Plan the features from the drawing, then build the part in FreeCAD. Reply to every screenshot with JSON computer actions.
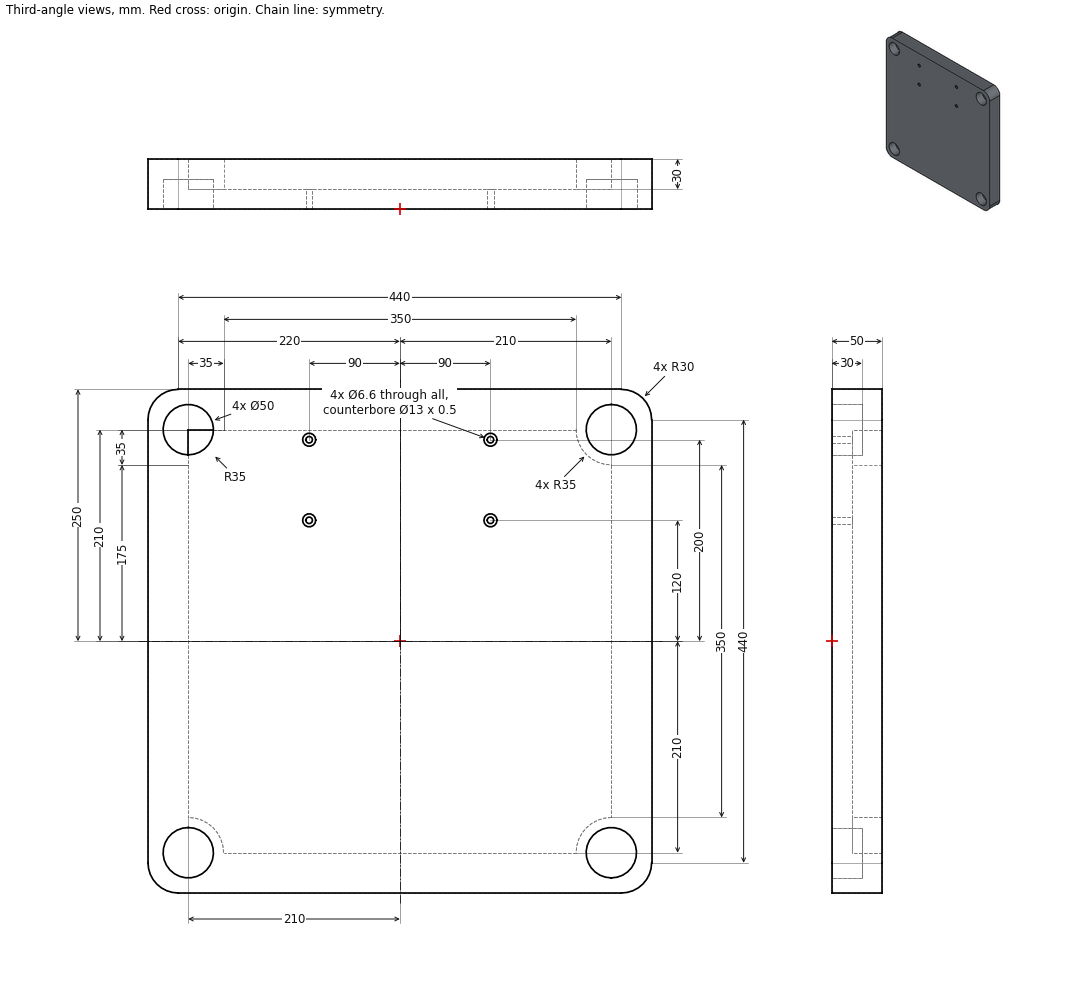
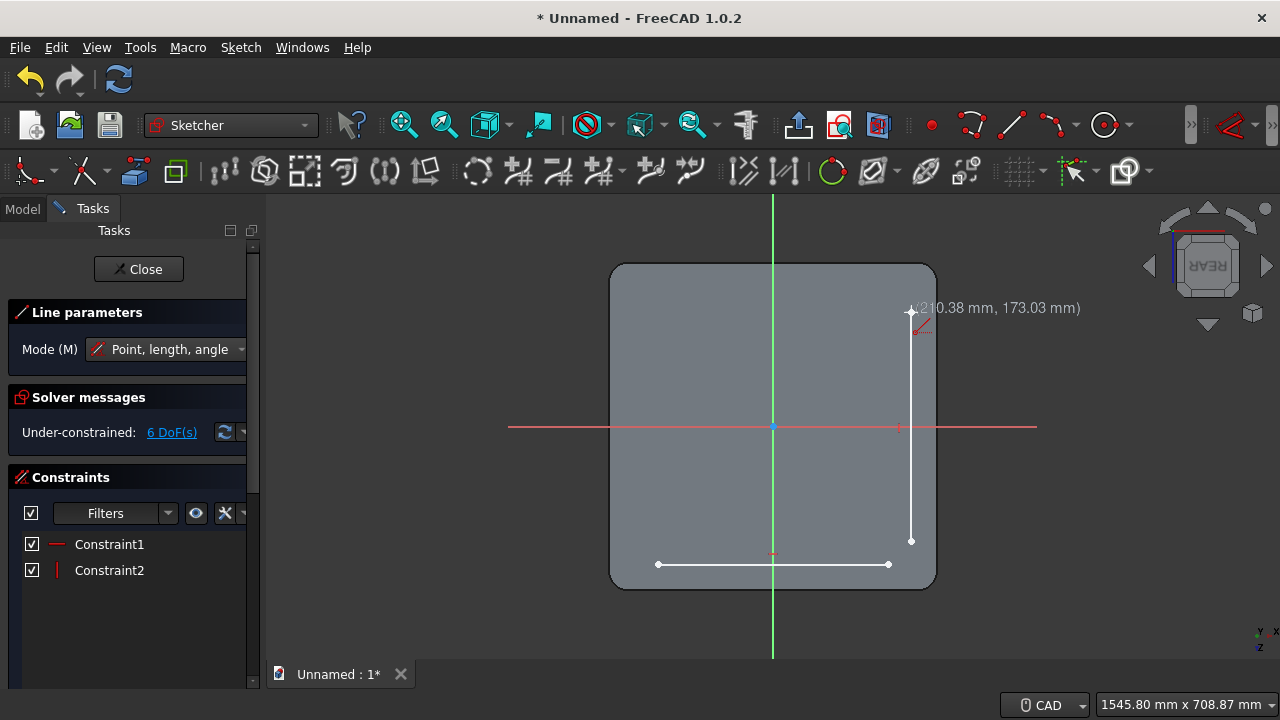
{"action": "left_click", "coordinate": [888, 289]}
{"action": "left_click", "coordinate": [658, 289]}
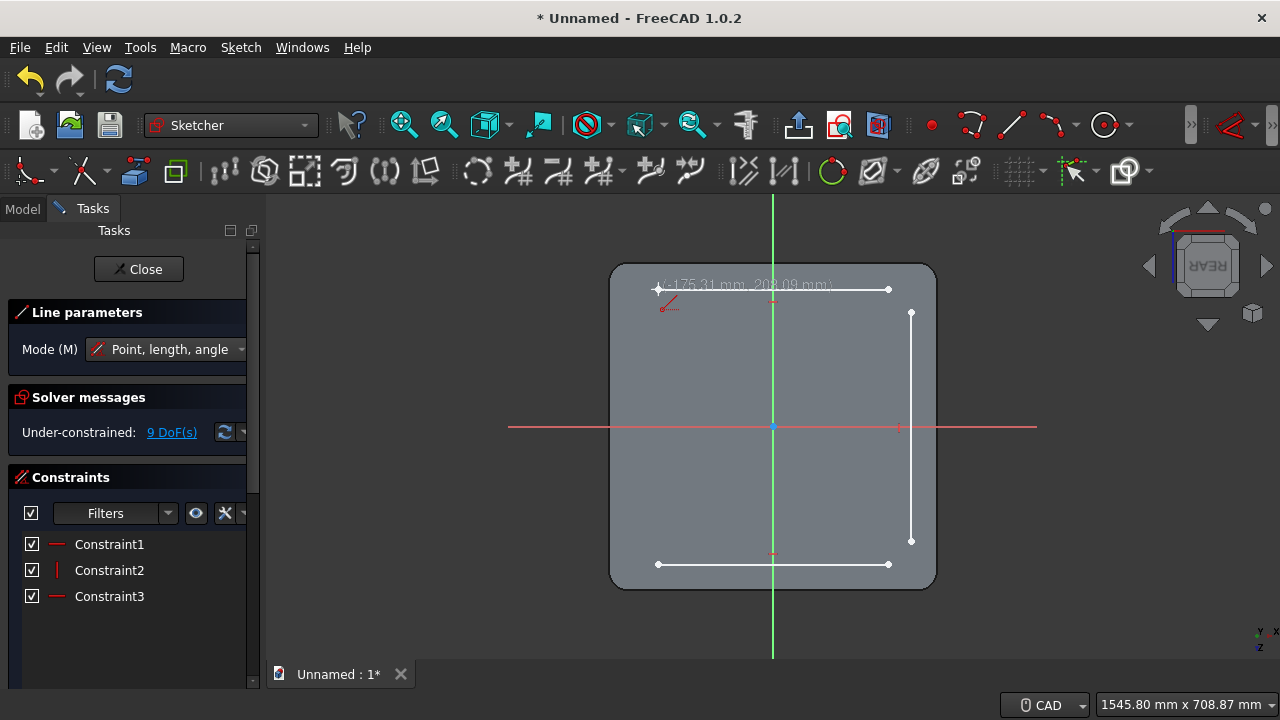
{"action": "left_click", "coordinate": [635, 312]}
{"action": "left_click", "coordinate": [635, 541]}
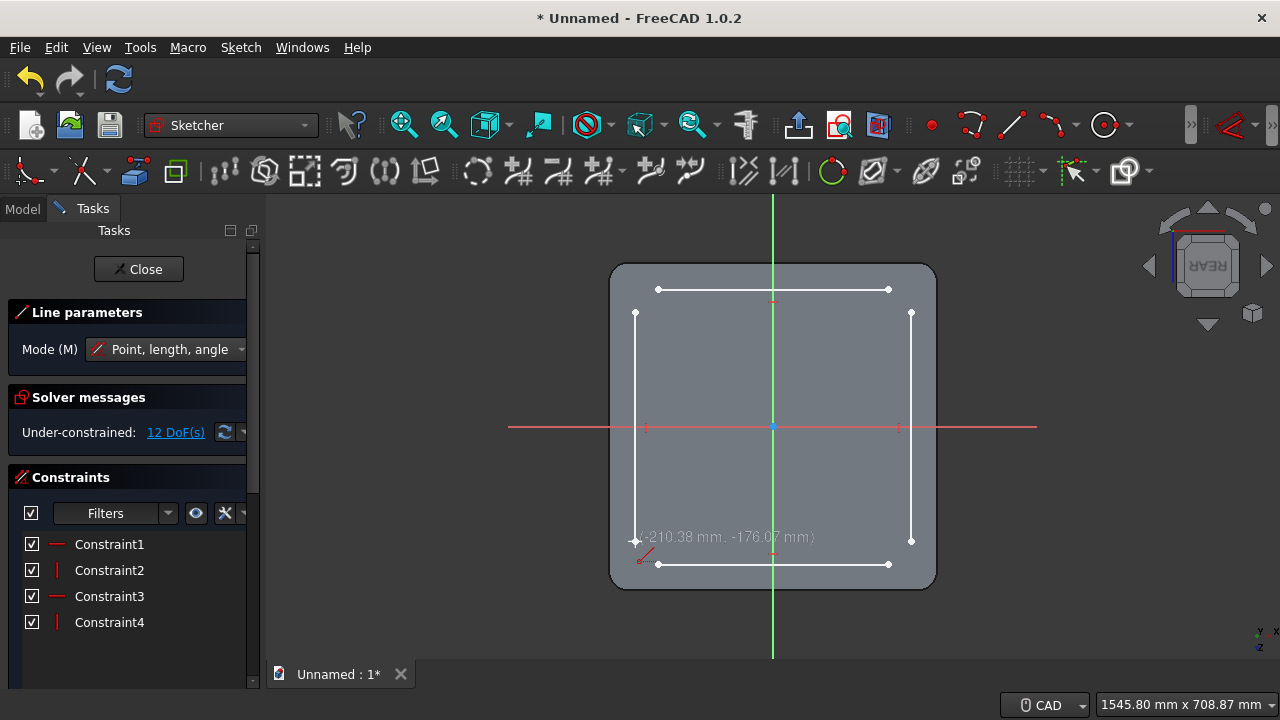
{"action": "key", "text": "g 3 a"}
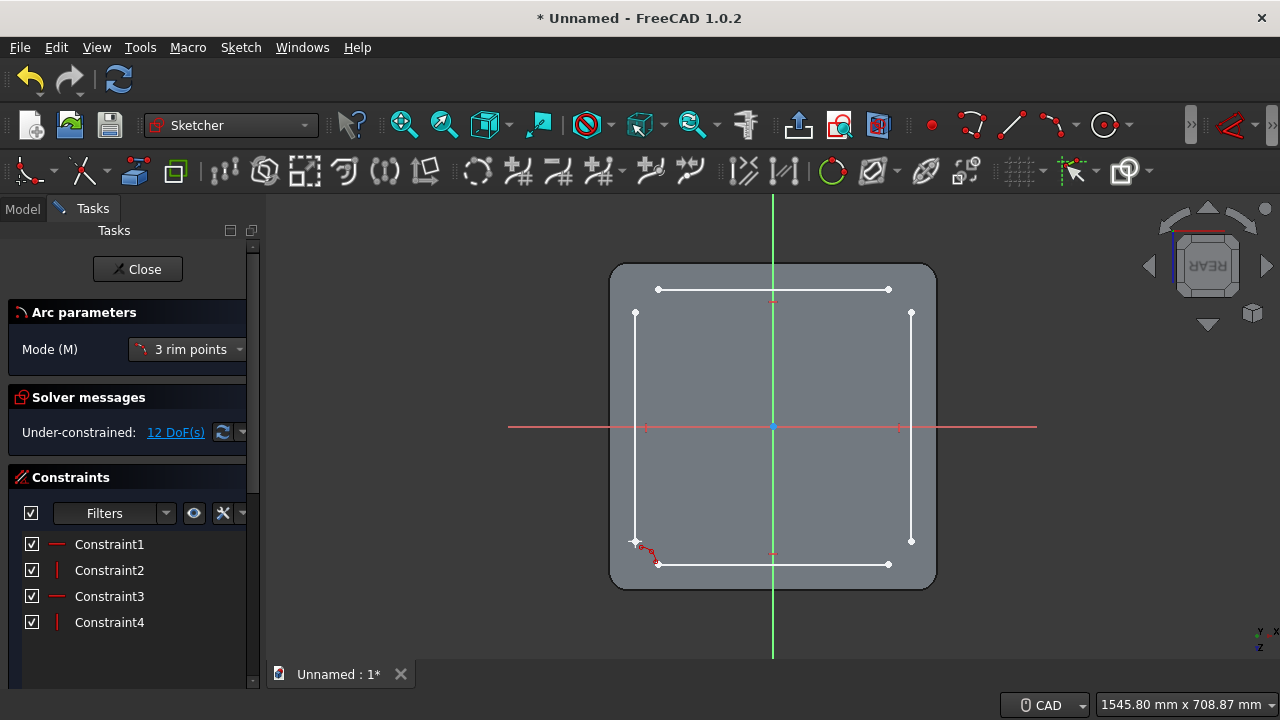
{"action": "left_click", "coordinate": [888, 565]}
{"action": "left_click", "coordinate": [911, 542]}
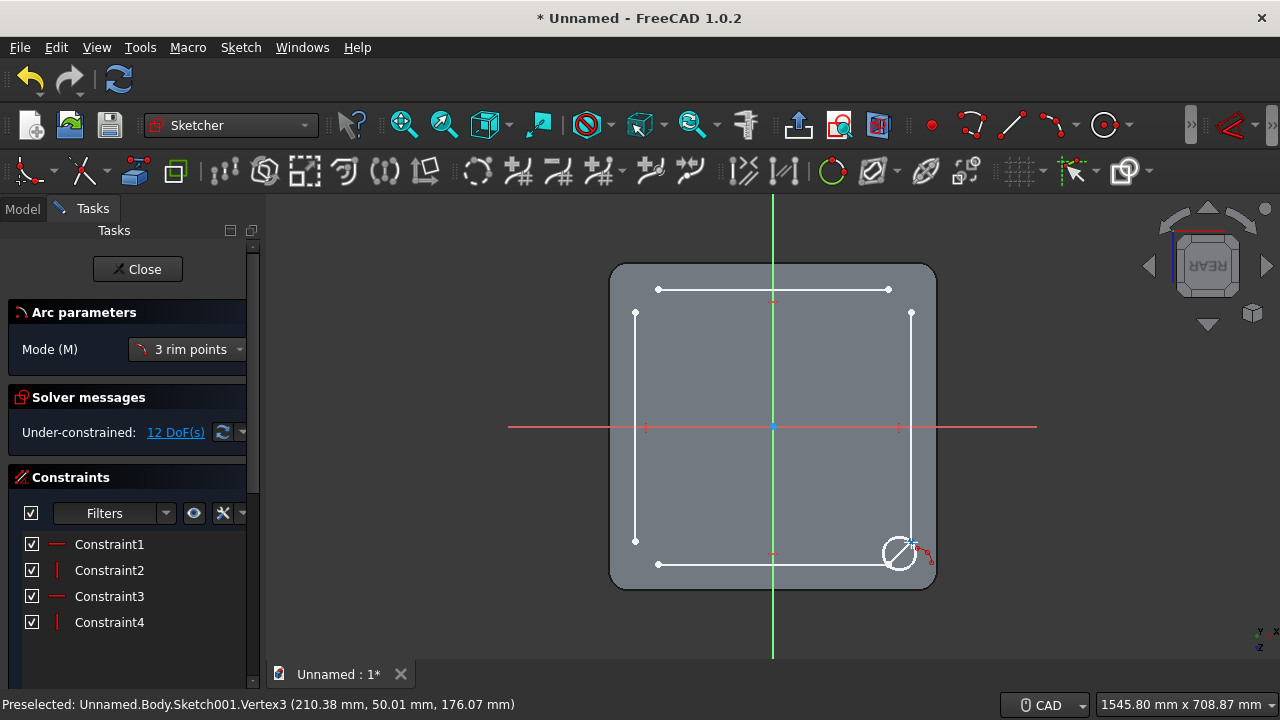
{"action": "scroll", "coordinate": [895, 548], "scroll_direction": "up", "scroll_amount": 5}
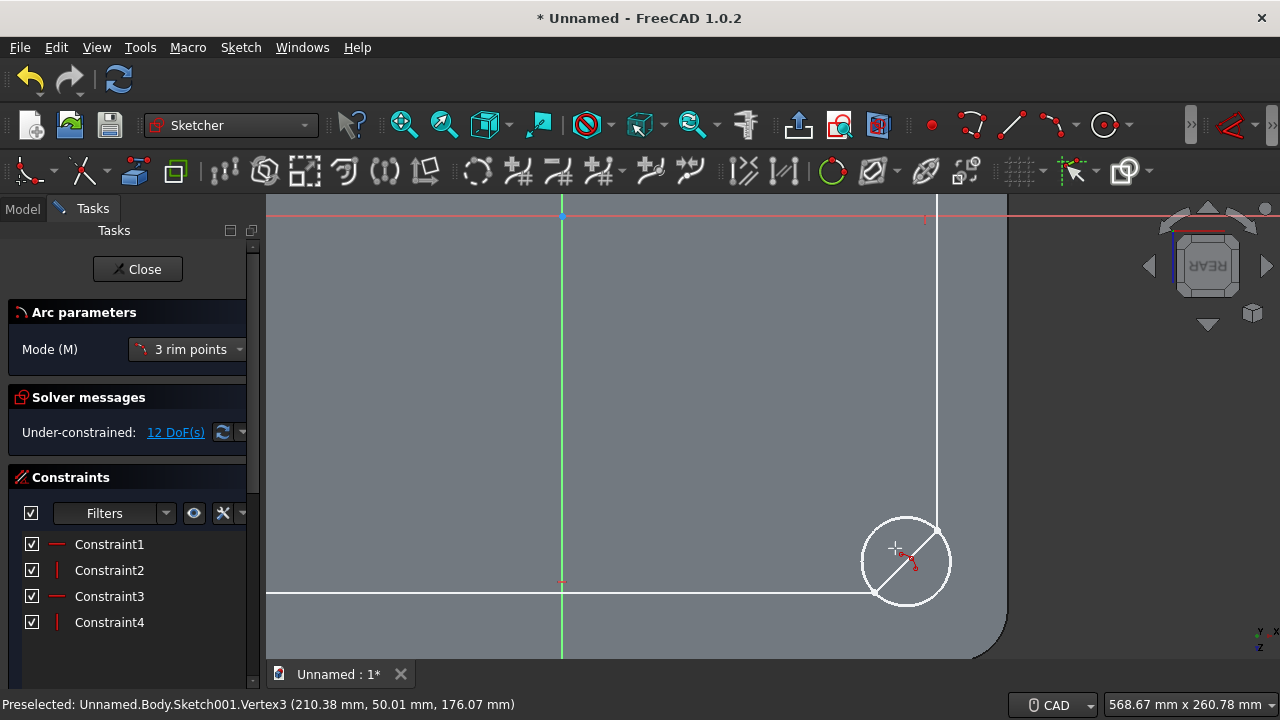
{"action": "left_click", "coordinate": [893, 547]}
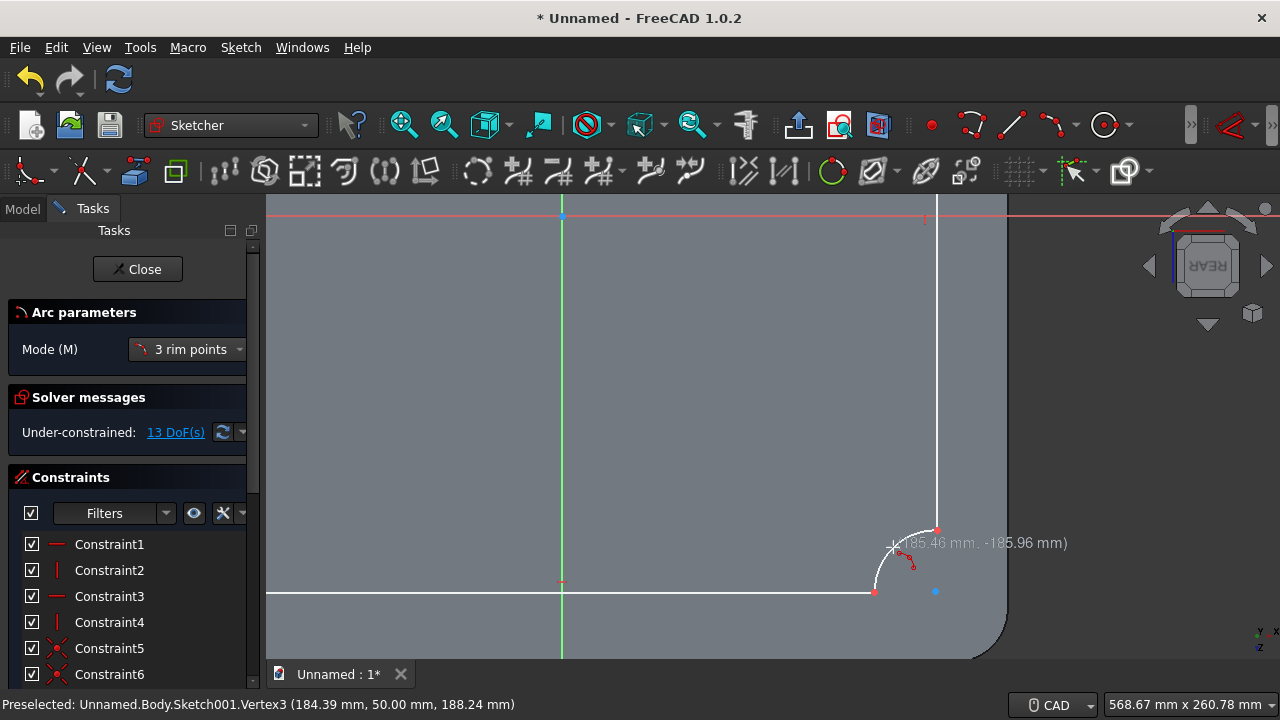
{"action": "scroll", "coordinate": [787, 549], "scroll_direction": "down", "scroll_amount": 5}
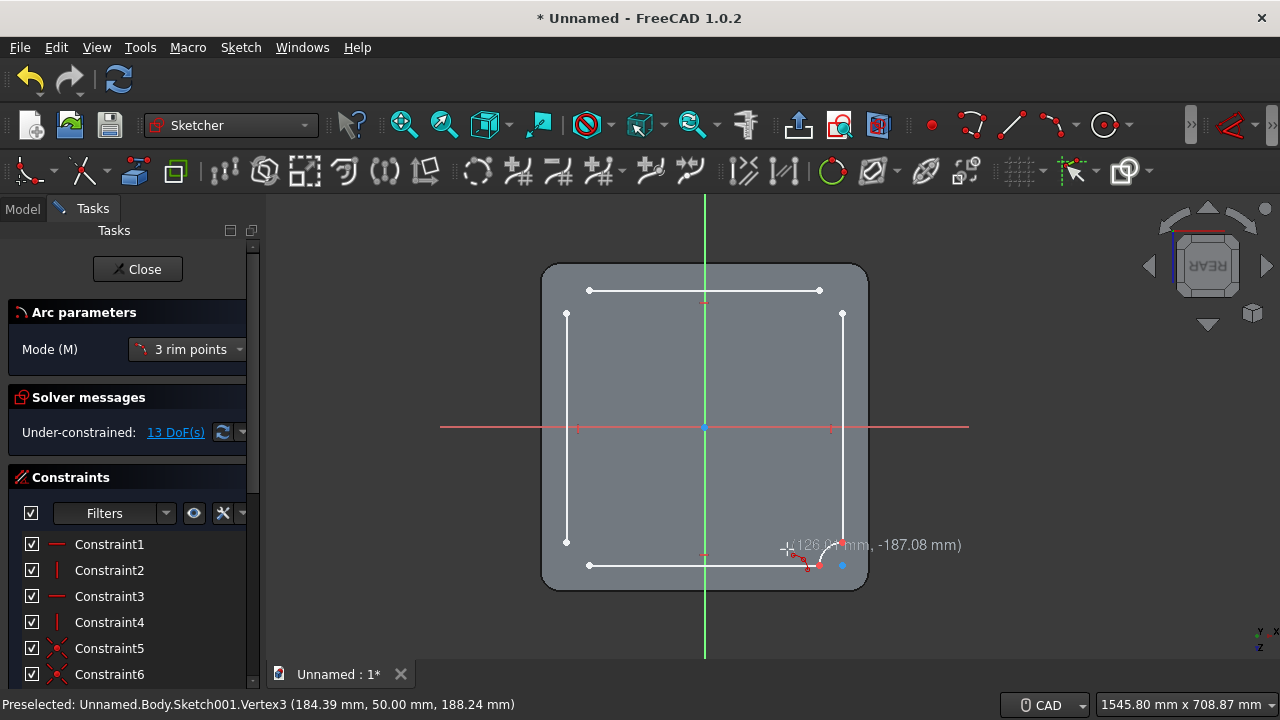
{"action": "left_click", "coordinate": [843, 314]}
{"action": "left_click", "coordinate": [820, 291]}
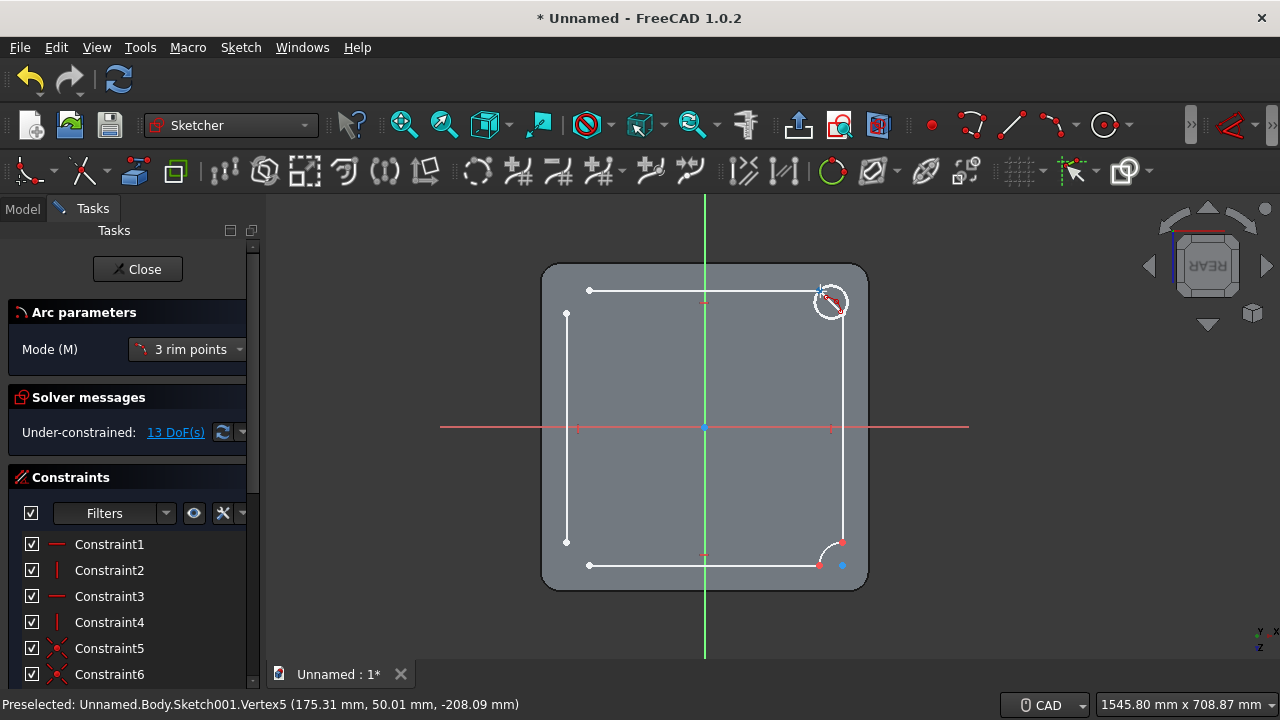
{"action": "scroll", "coordinate": [826, 306], "scroll_direction": "up", "scroll_amount": 5}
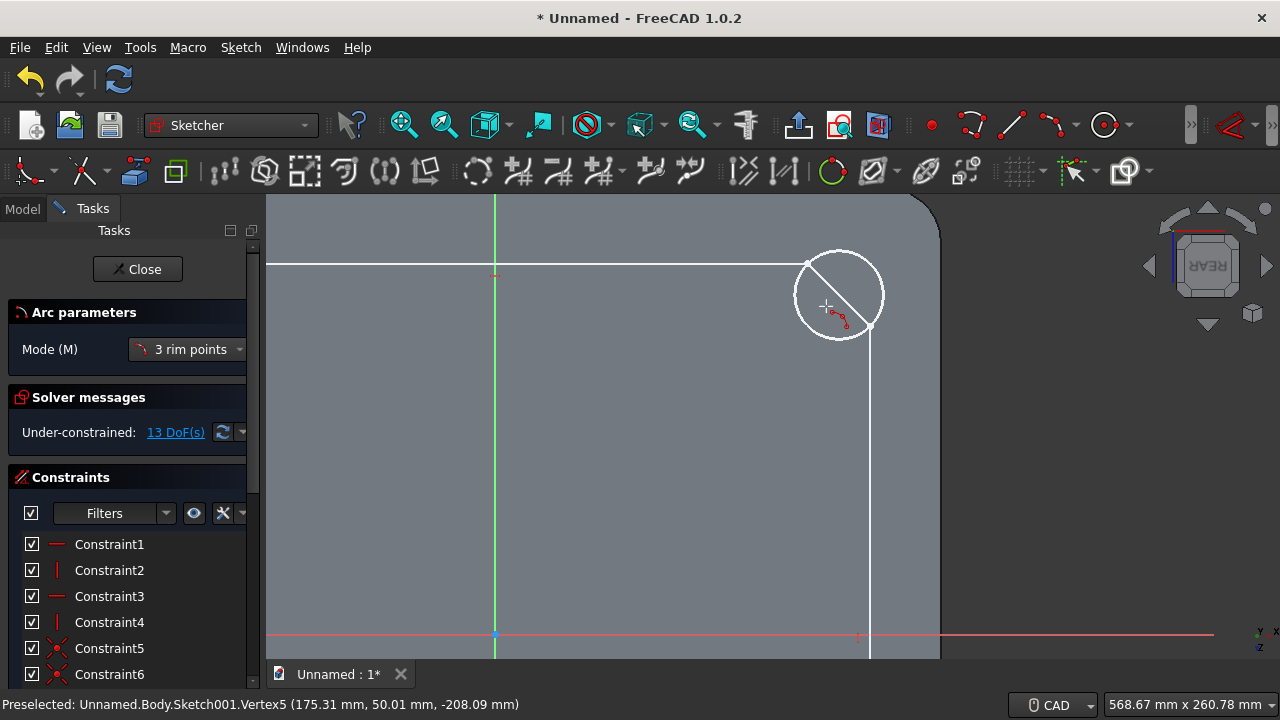
{"action": "left_click", "coordinate": [826, 305]}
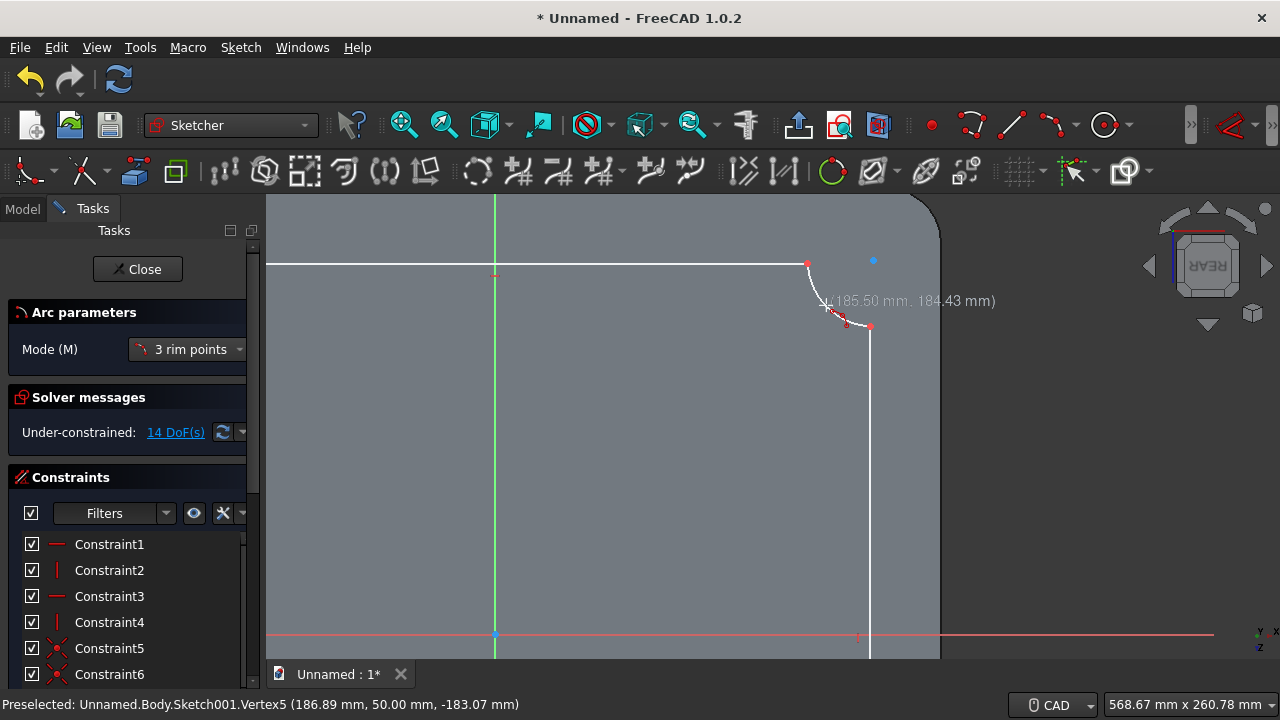
{"action": "scroll", "coordinate": [826, 305], "scroll_direction": "down", "scroll_amount": 5}